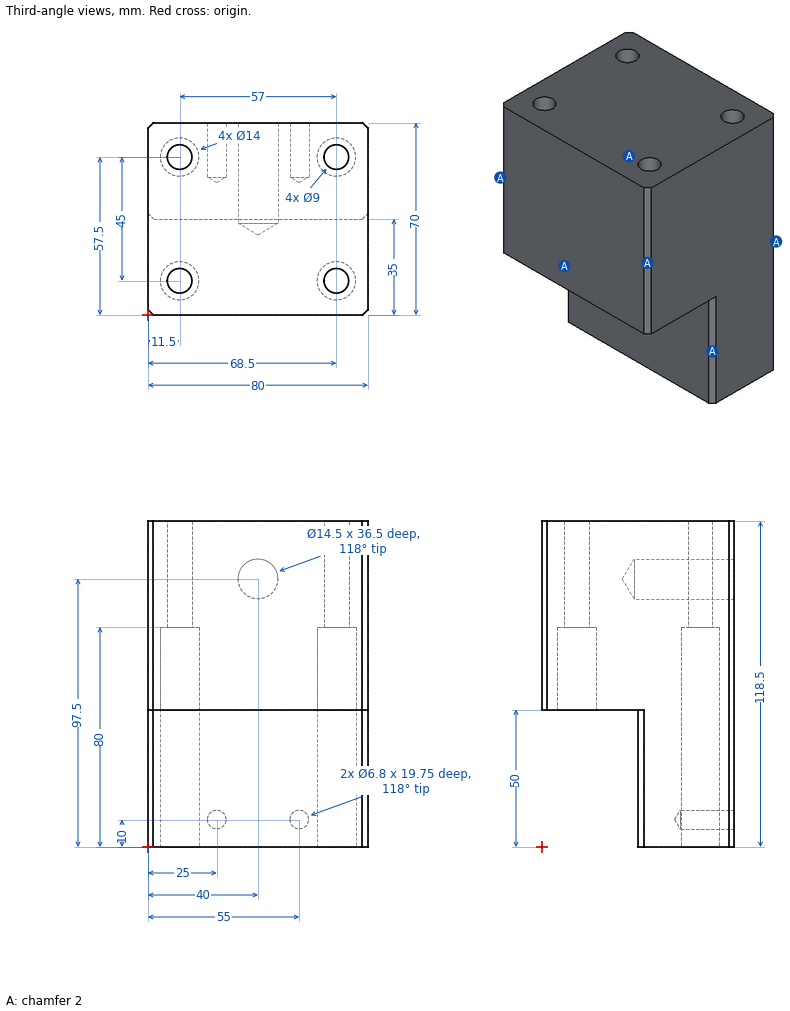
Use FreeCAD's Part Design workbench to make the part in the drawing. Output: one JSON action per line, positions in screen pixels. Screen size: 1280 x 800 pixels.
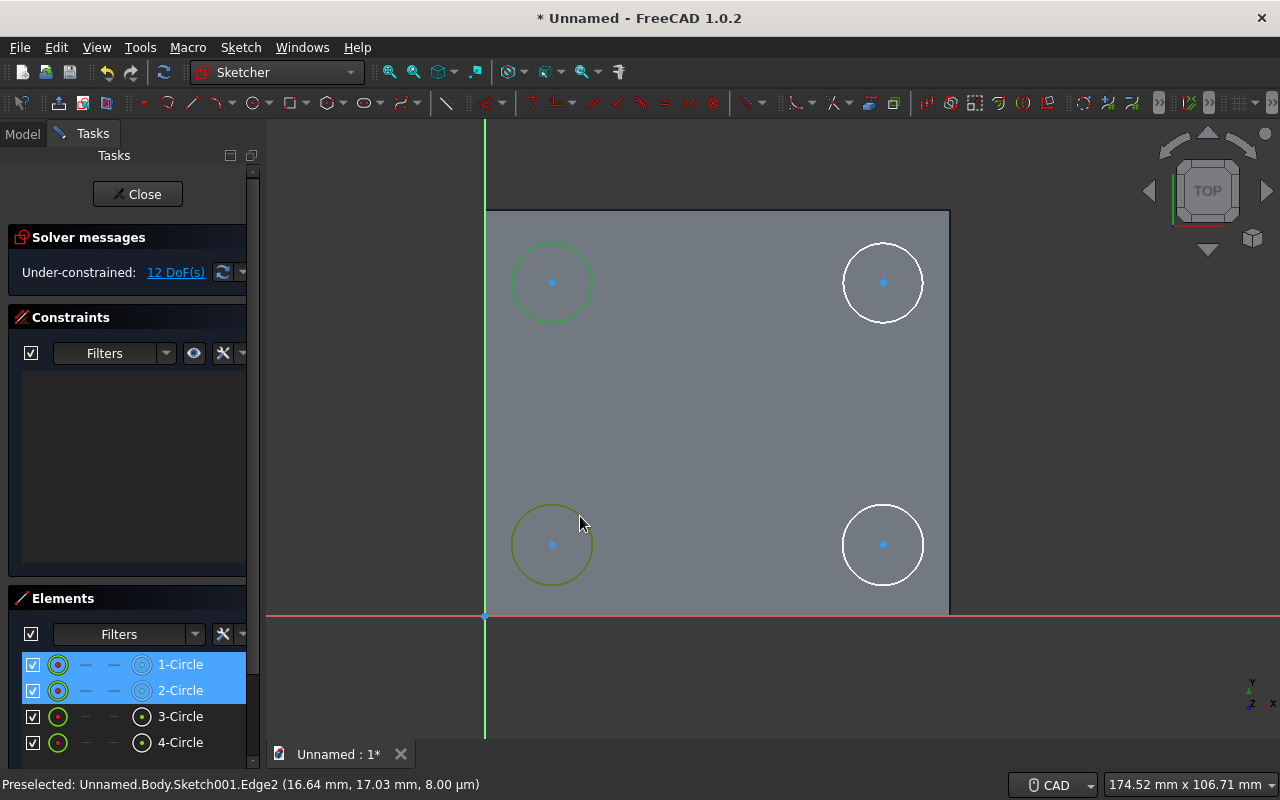
{"action": "left_click", "coordinate": [911, 255]}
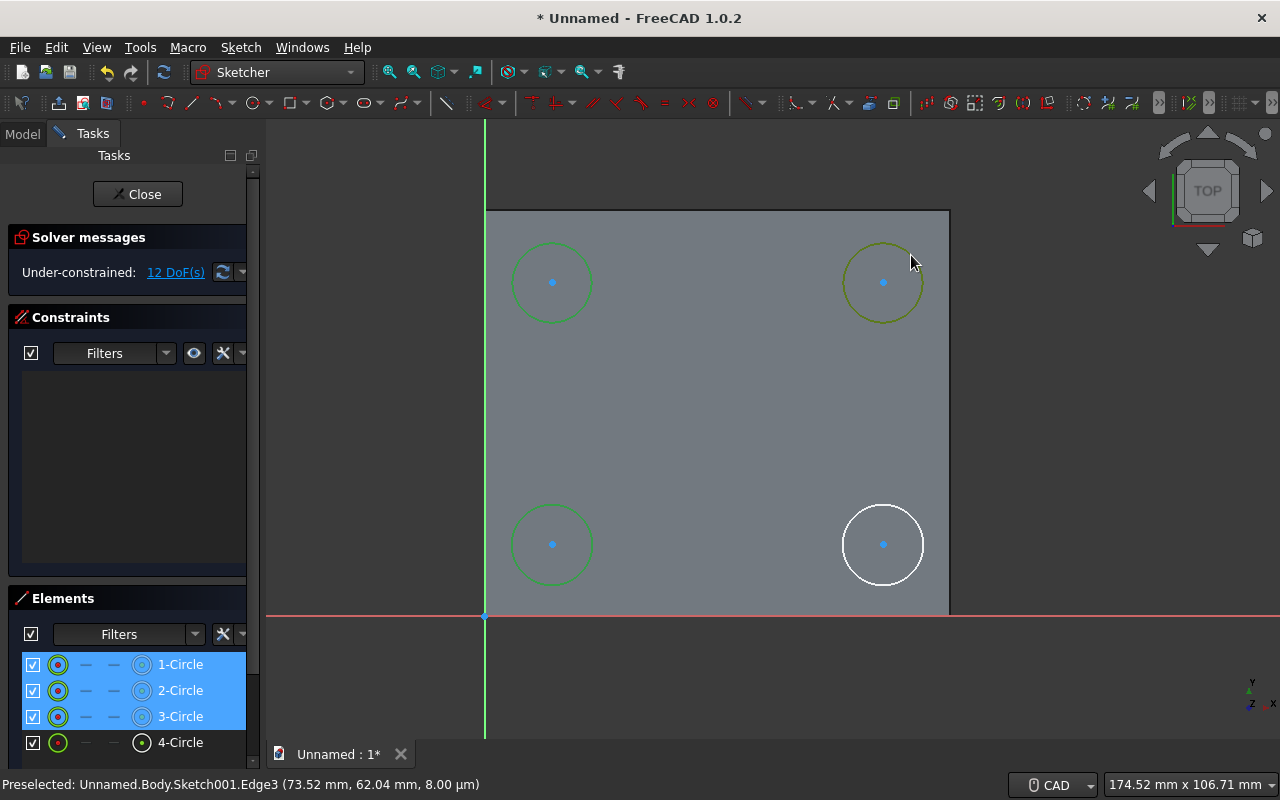
{"action": "left_click", "coordinate": [911, 516]}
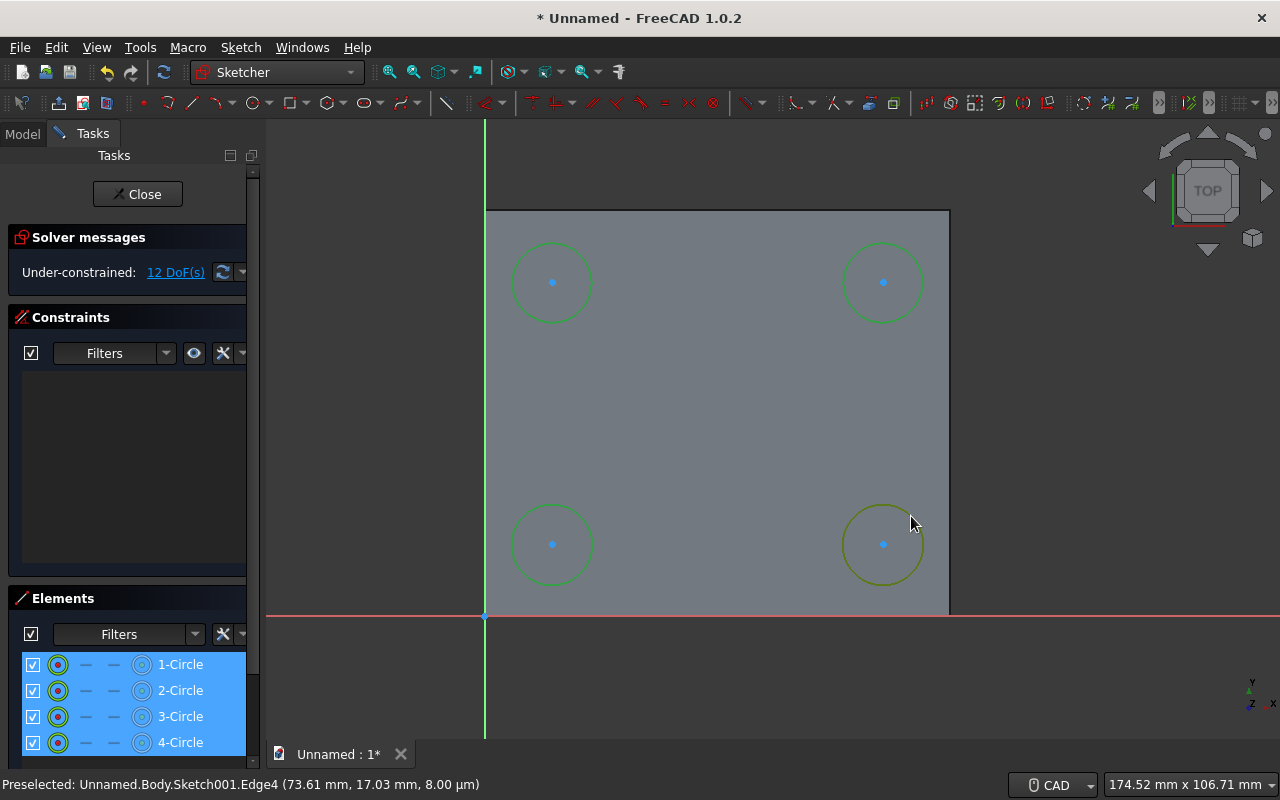
{"action": "key", "text": "e"}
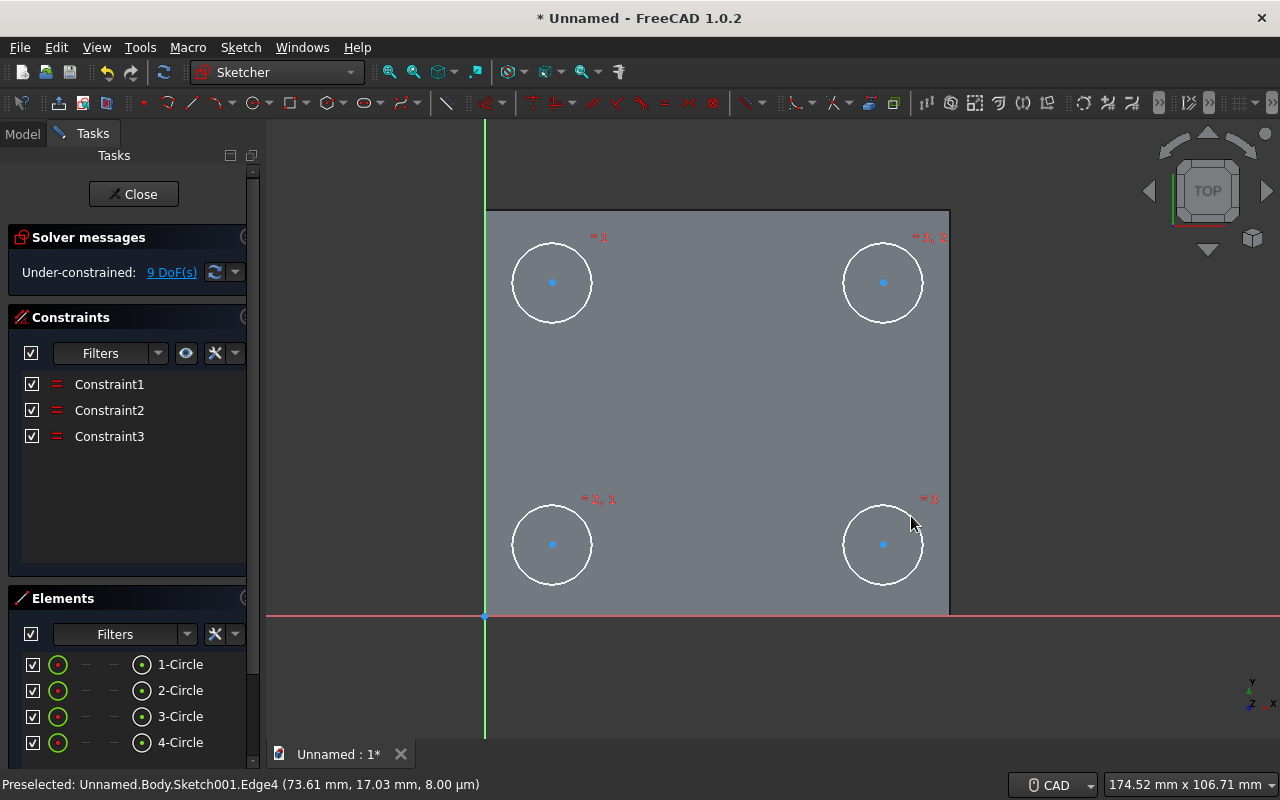
{"action": "left_click", "coordinate": [552, 283]}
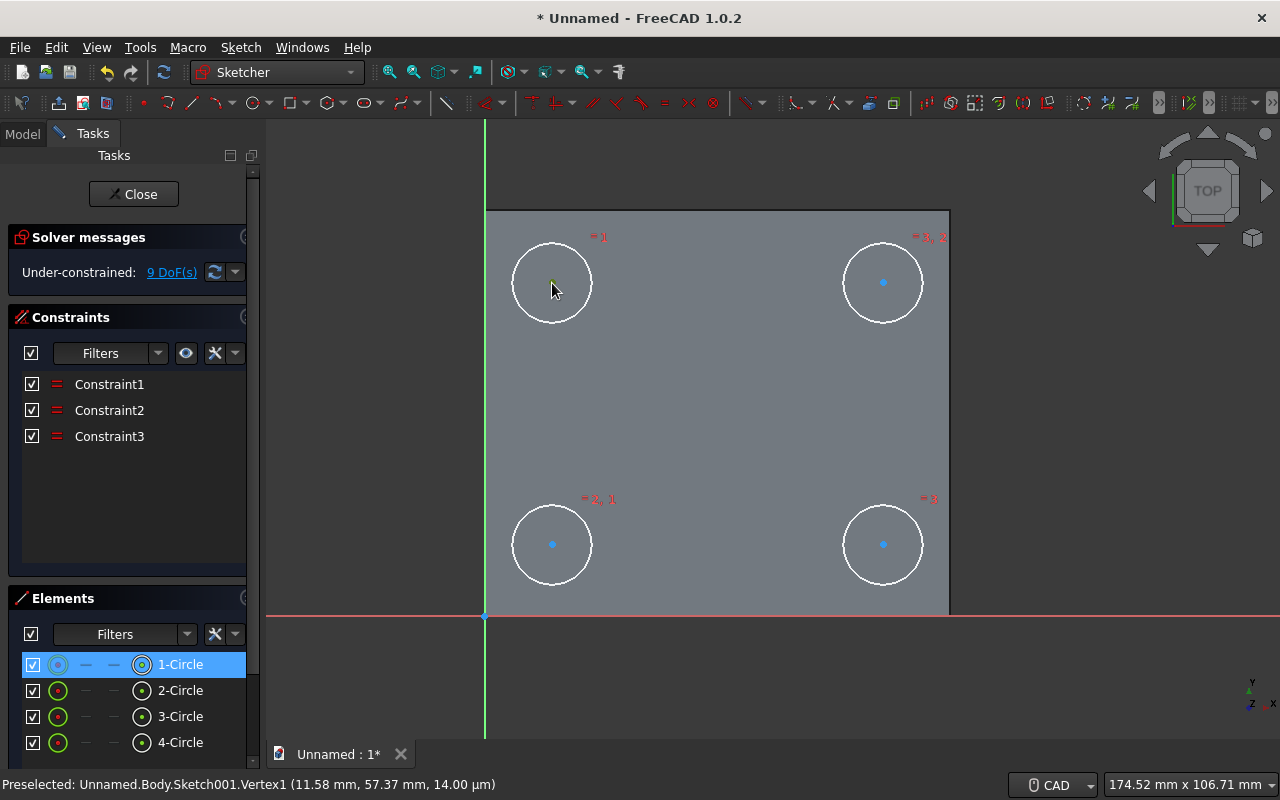
{"action": "left_click", "coordinate": [552, 545]}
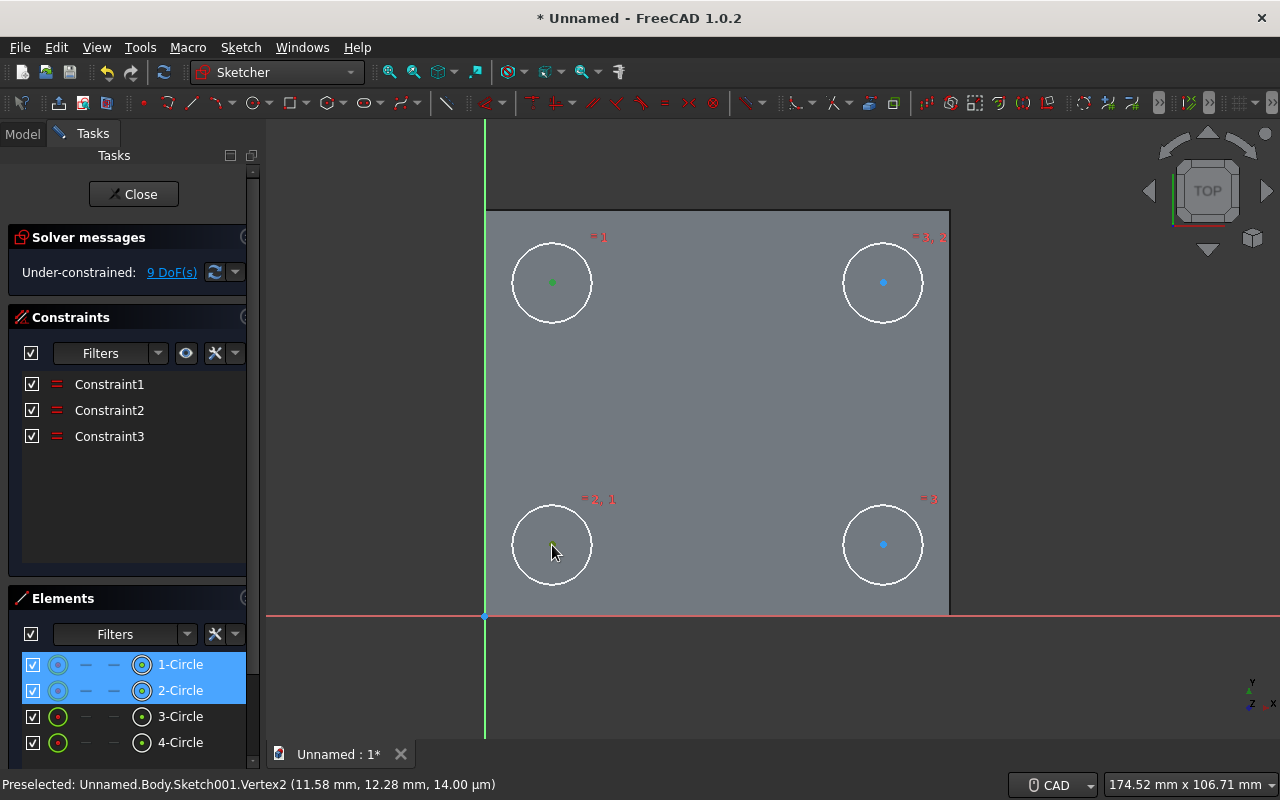
{"action": "key", "text": "v"}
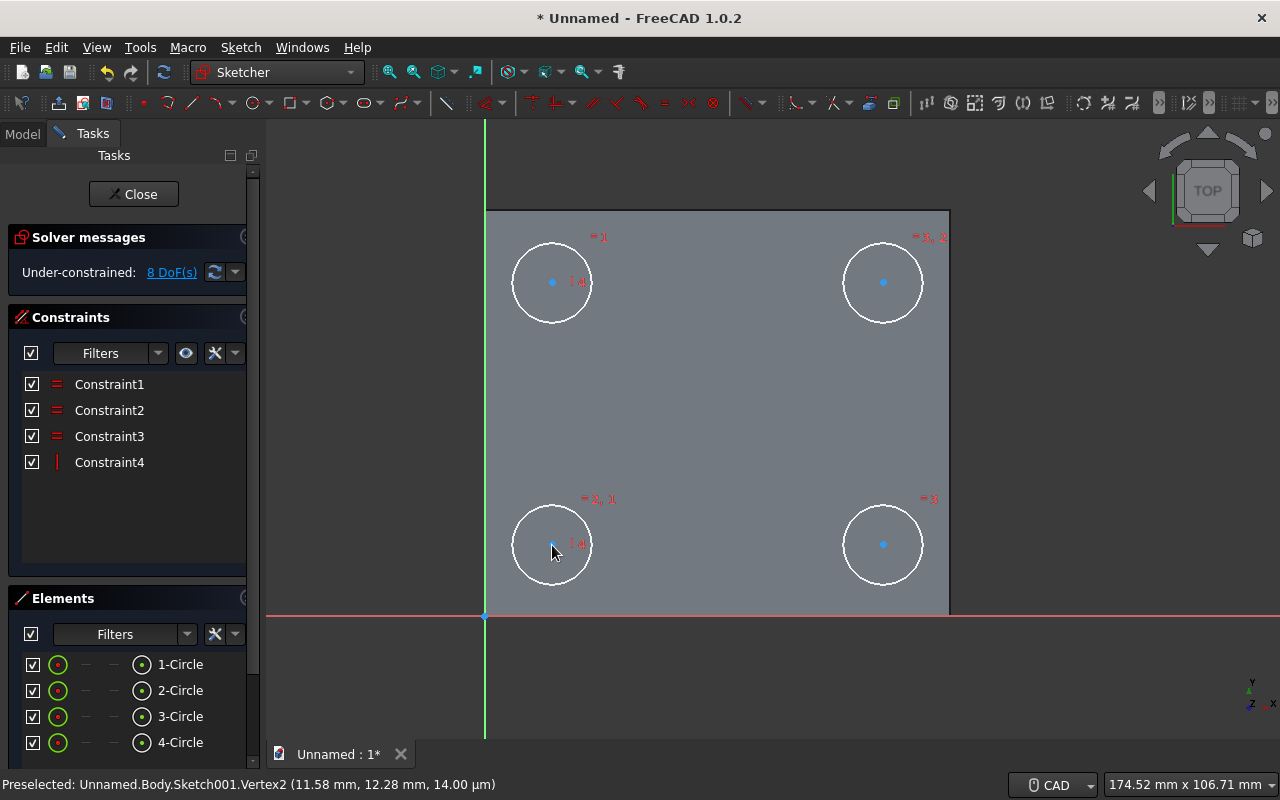
{"action": "left_click", "coordinate": [552, 283]}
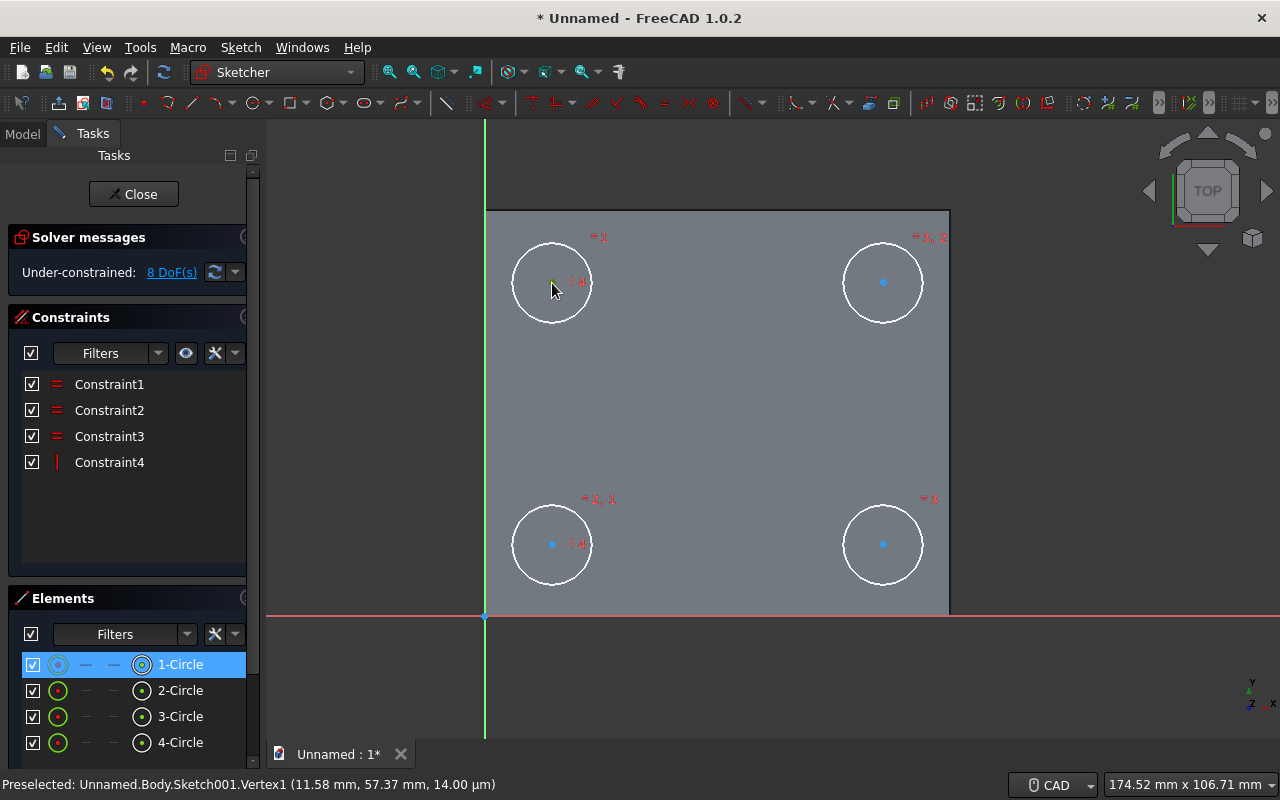
{"action": "left_click", "coordinate": [883, 283]}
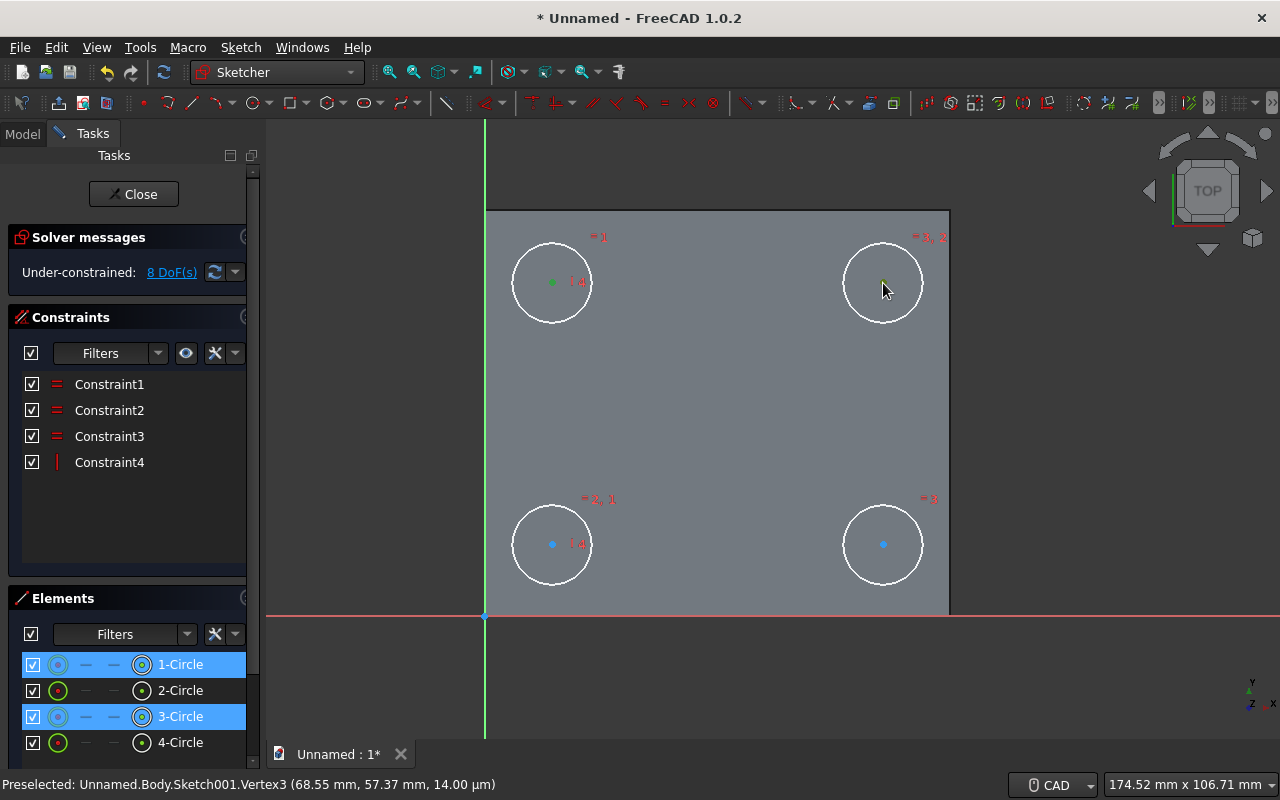
{"action": "left_click", "coordinate": [574, 104]}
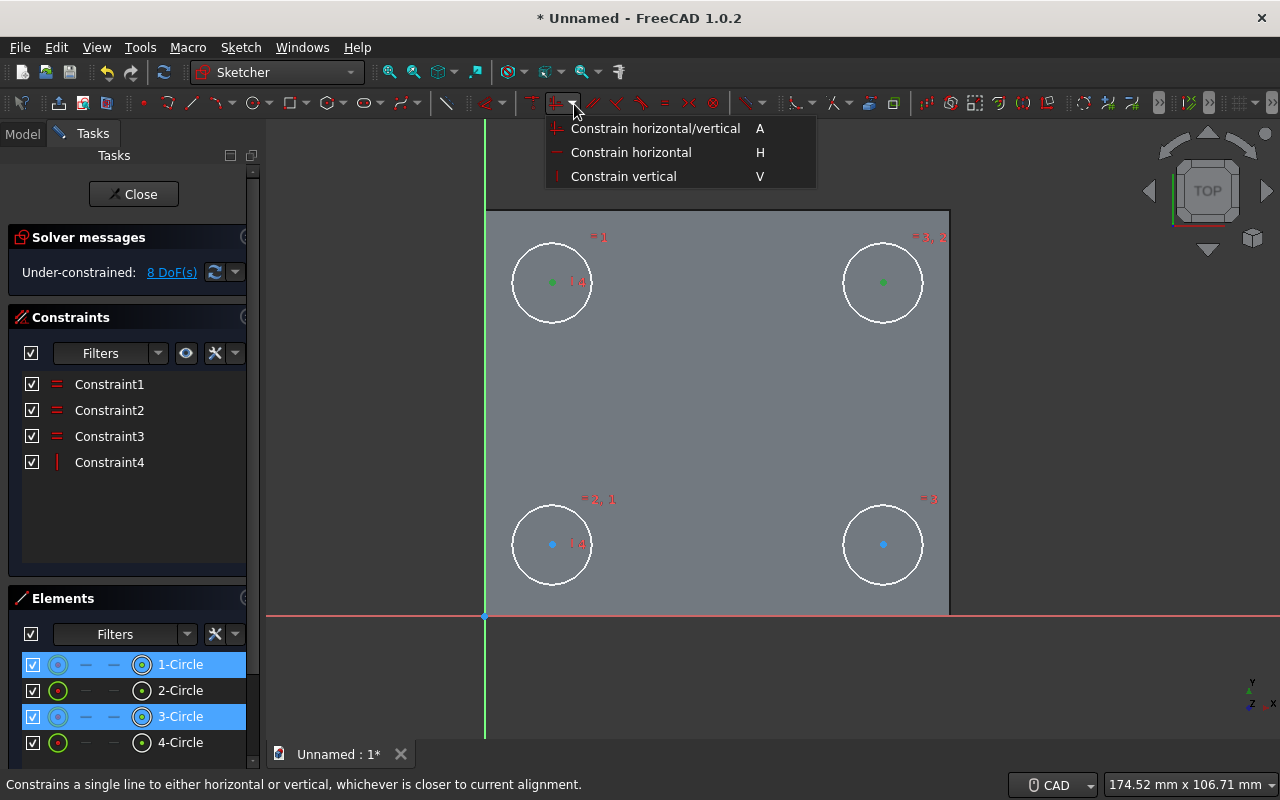
{"action": "left_click", "coordinate": [681, 152]}